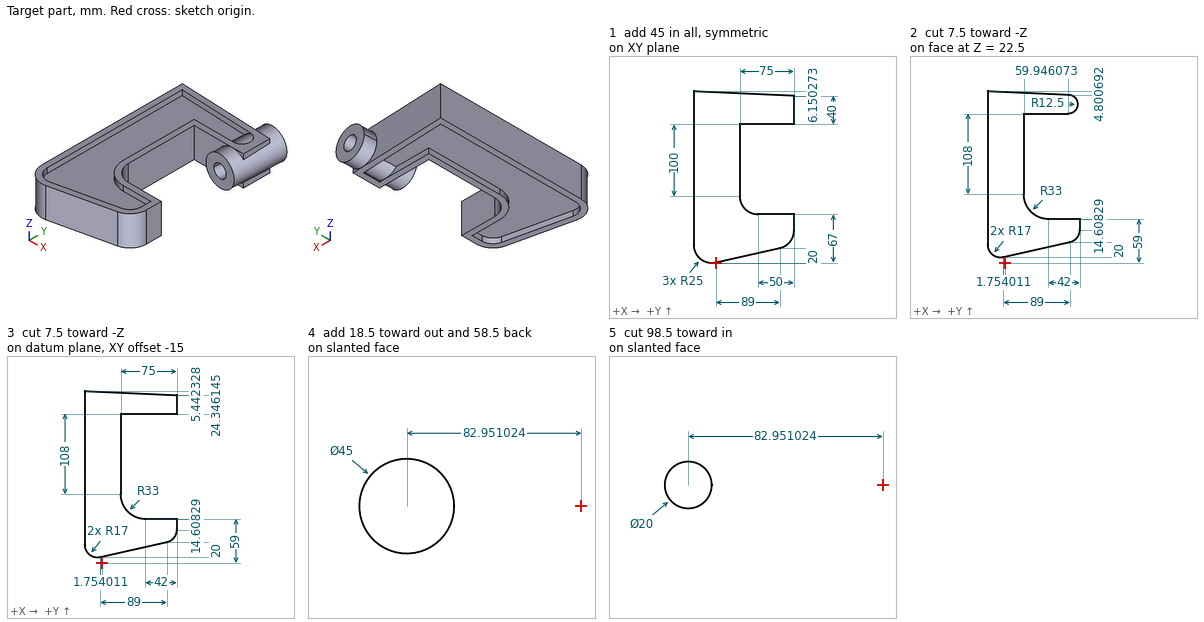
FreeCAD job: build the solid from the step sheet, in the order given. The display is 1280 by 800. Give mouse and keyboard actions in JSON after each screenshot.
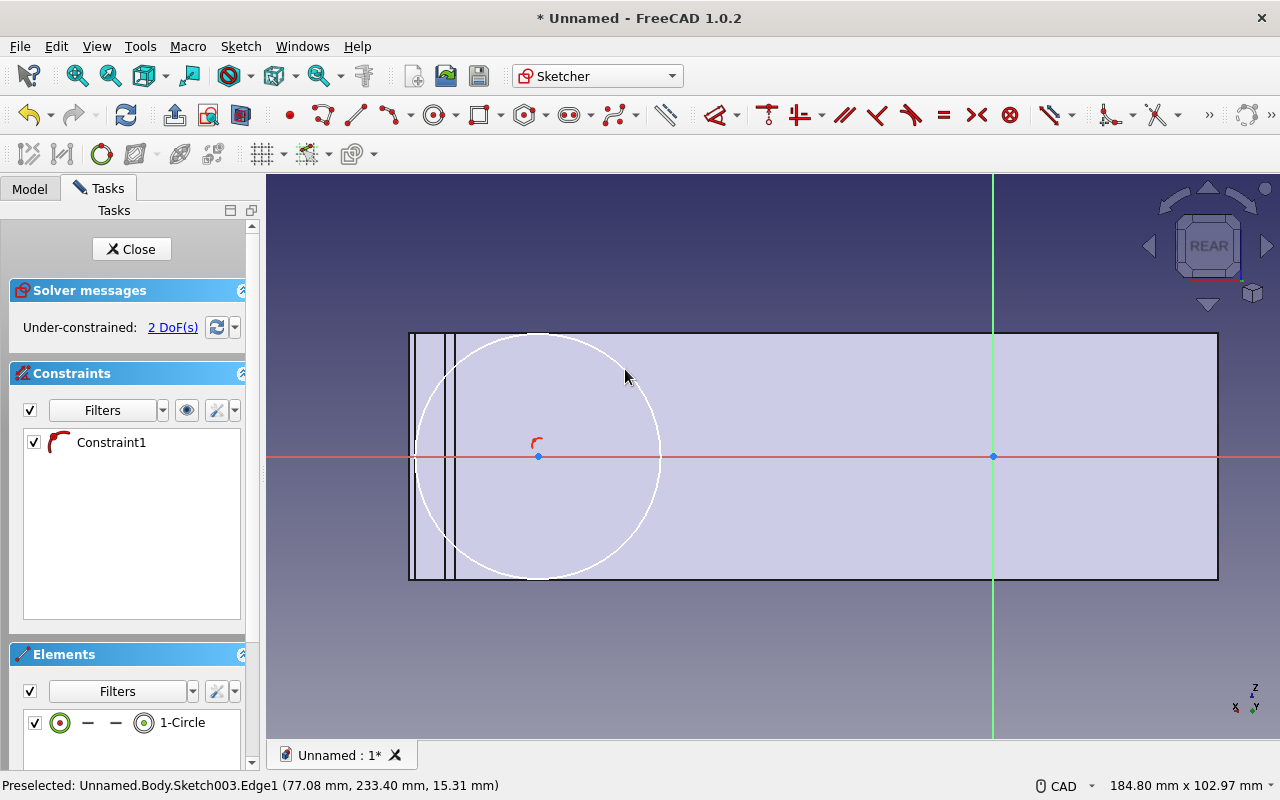
{"action": "left_click", "coordinate": [714, 116]}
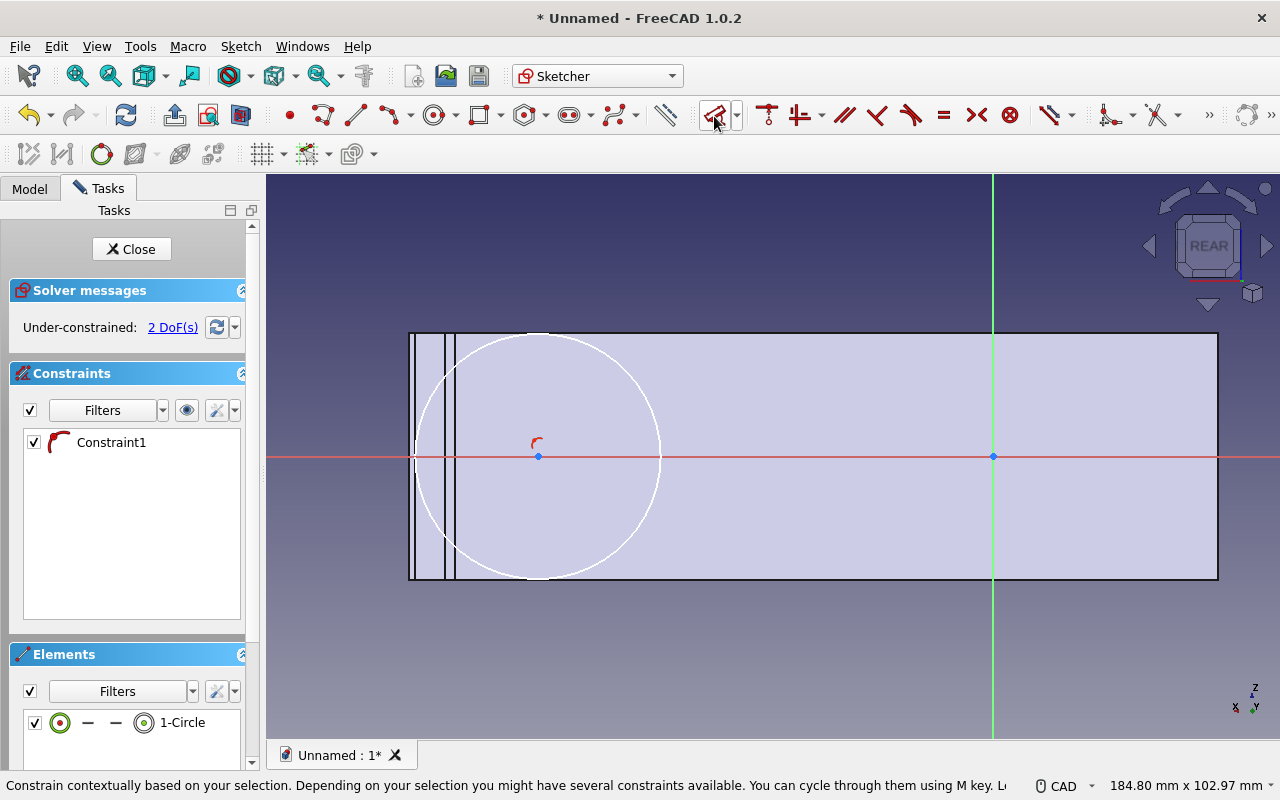
{"action": "left_click", "coordinate": [624, 369]}
{"action": "left_click", "coordinate": [646, 346]}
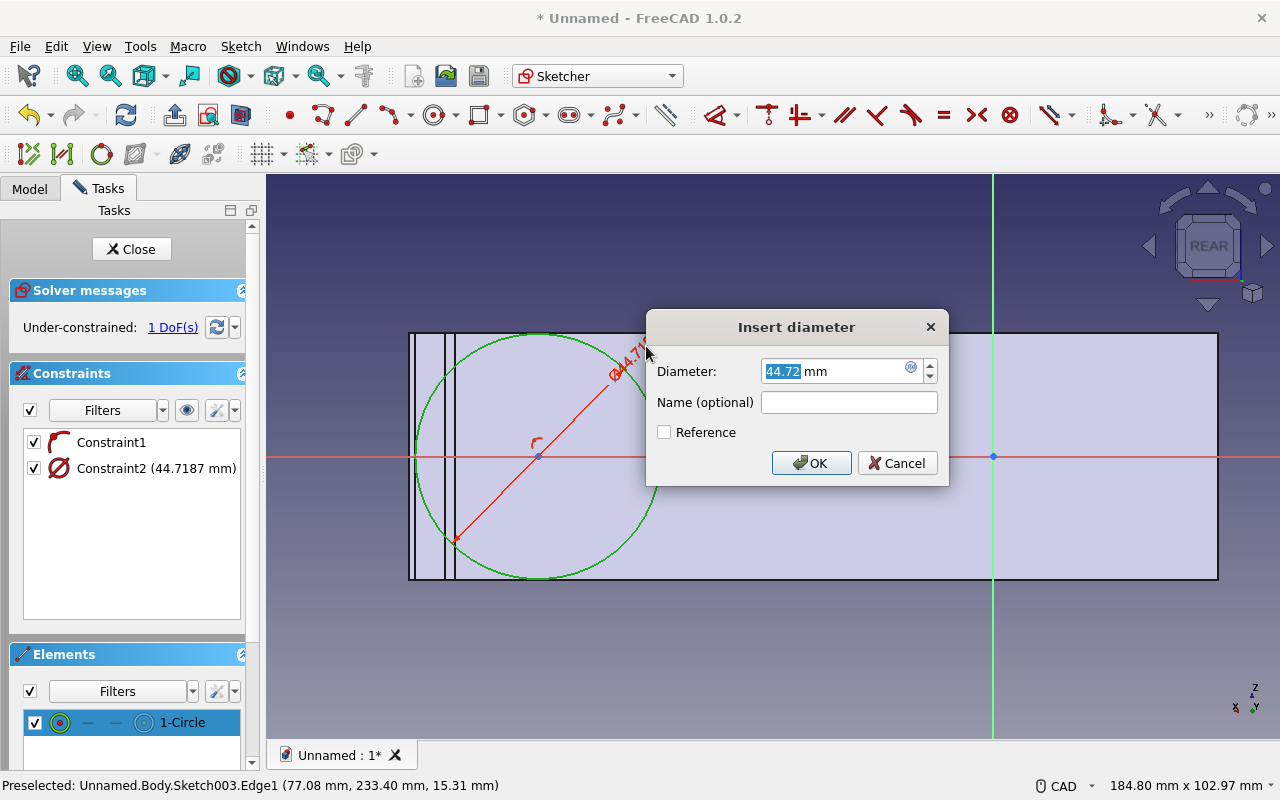
{"action": "type", "text": "45"}
{"action": "key", "text": "Return"}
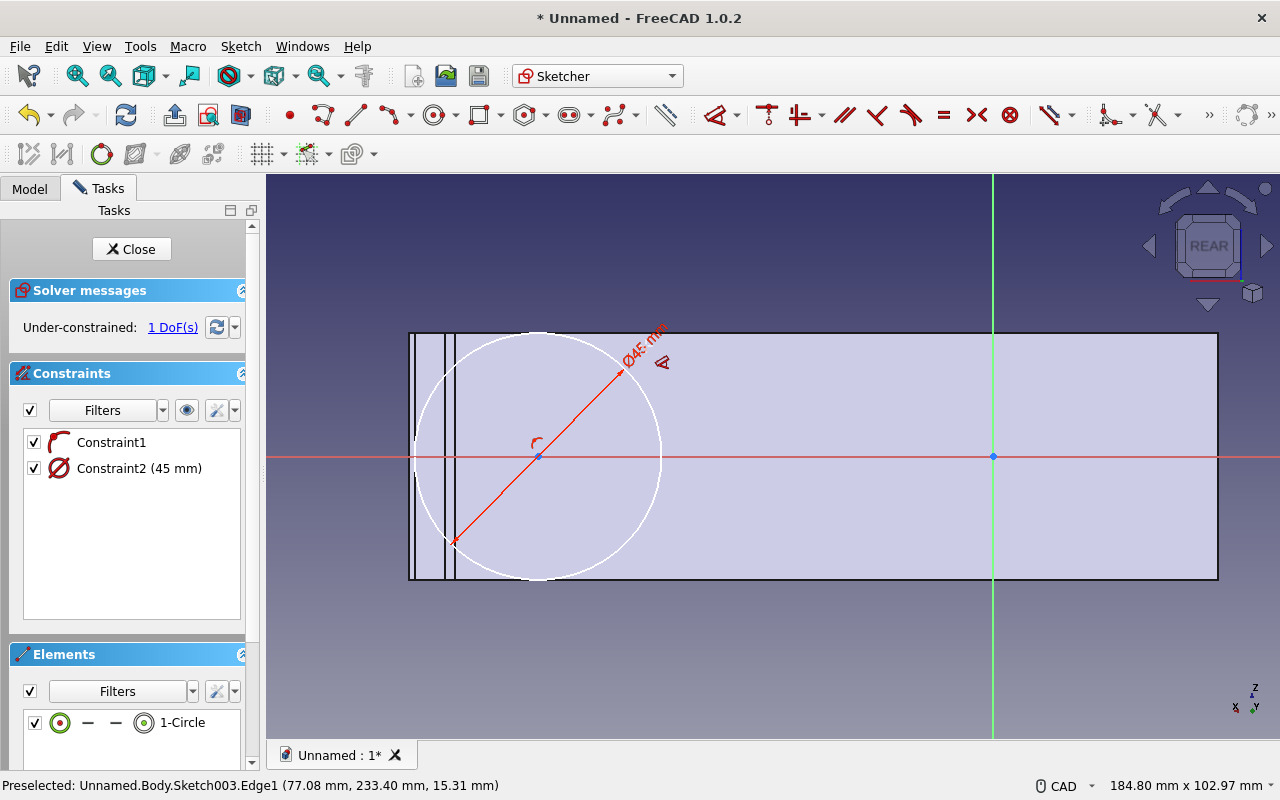
{"action": "left_click", "coordinate": [538, 456]}
{"action": "left_click", "coordinate": [766, 490]}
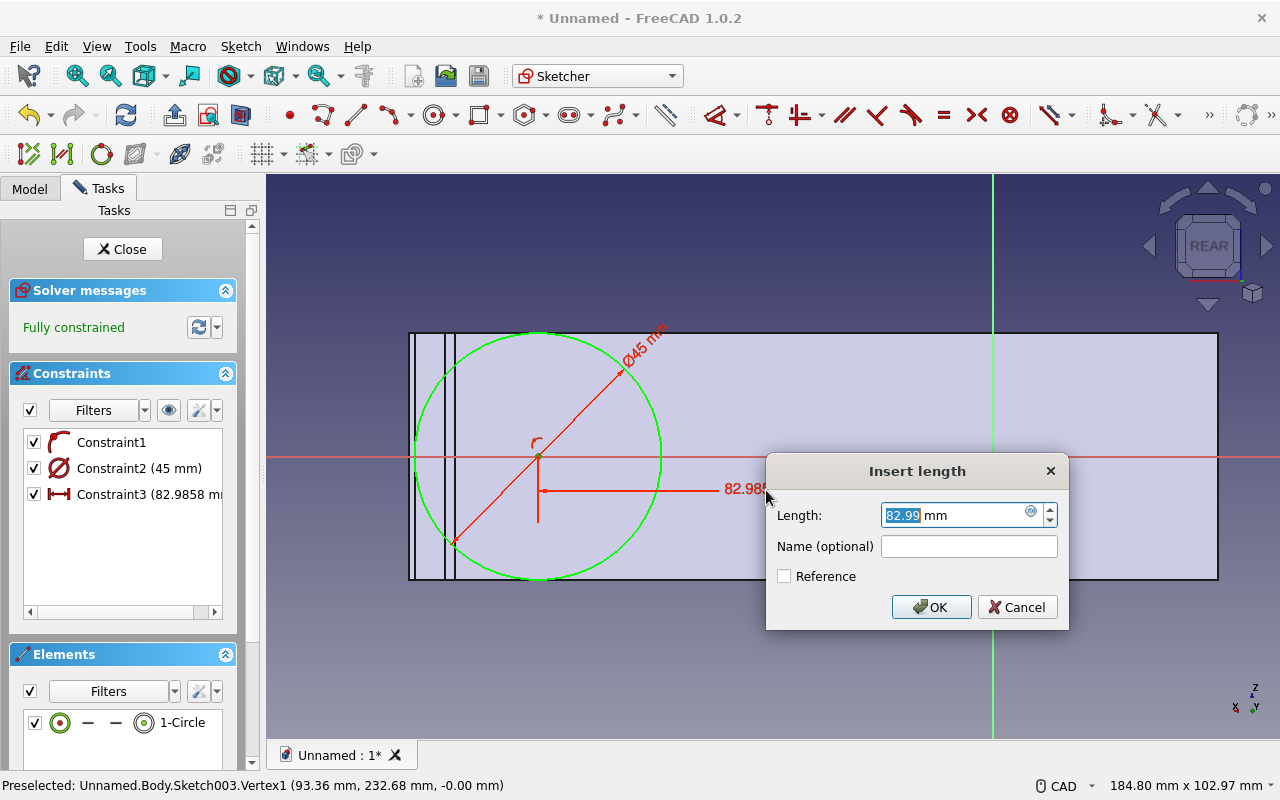
{"action": "type", "text": "82.951024"}
{"action": "key", "text": "Return"}
{"action": "key", "text": "Escape"}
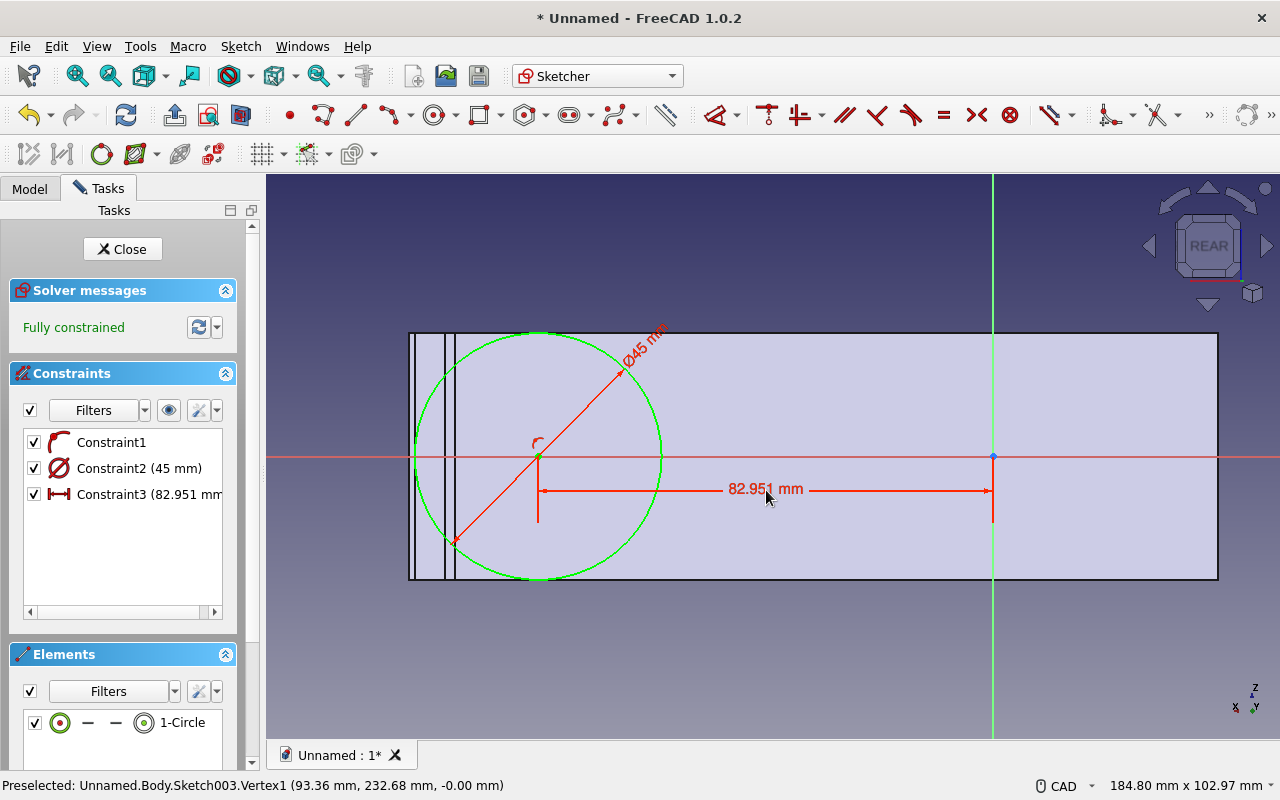
{"action": "left_click", "coordinate": [123, 249]}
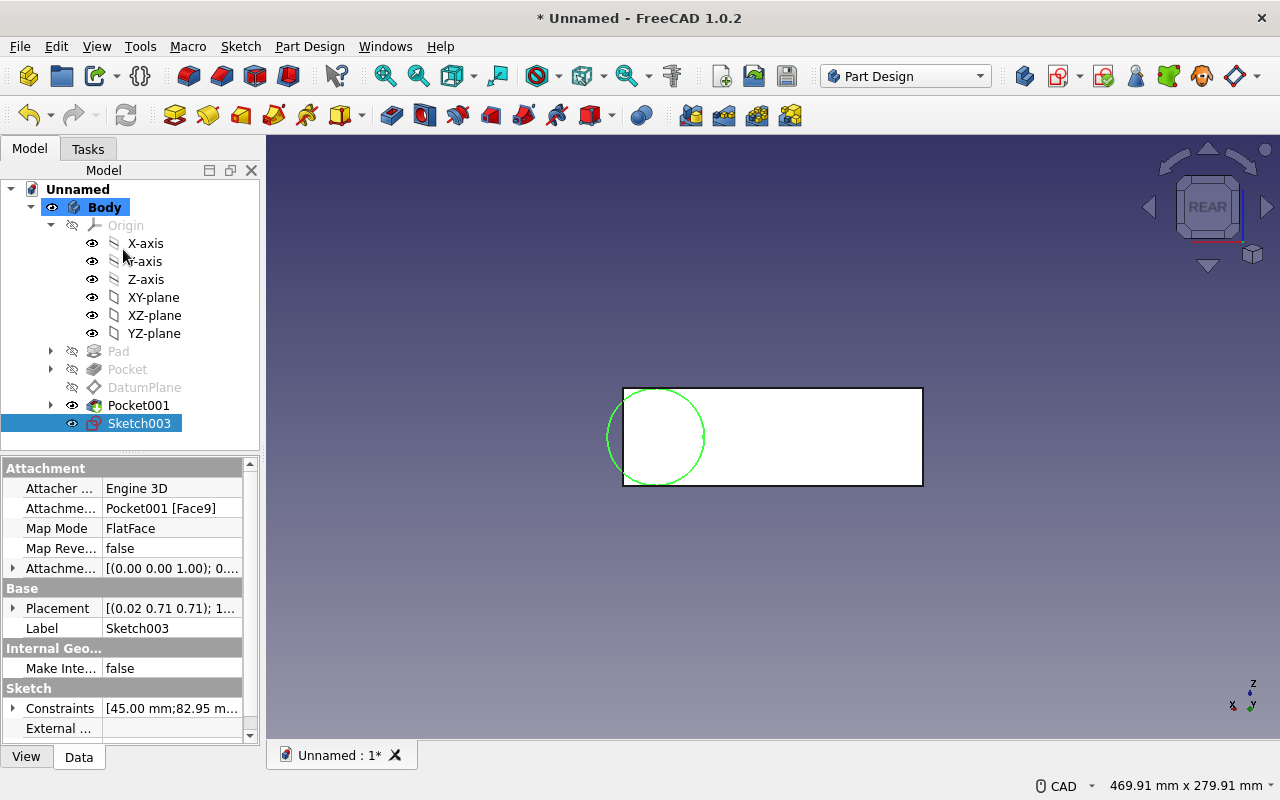
{"action": "left_click", "coordinate": [175, 116]}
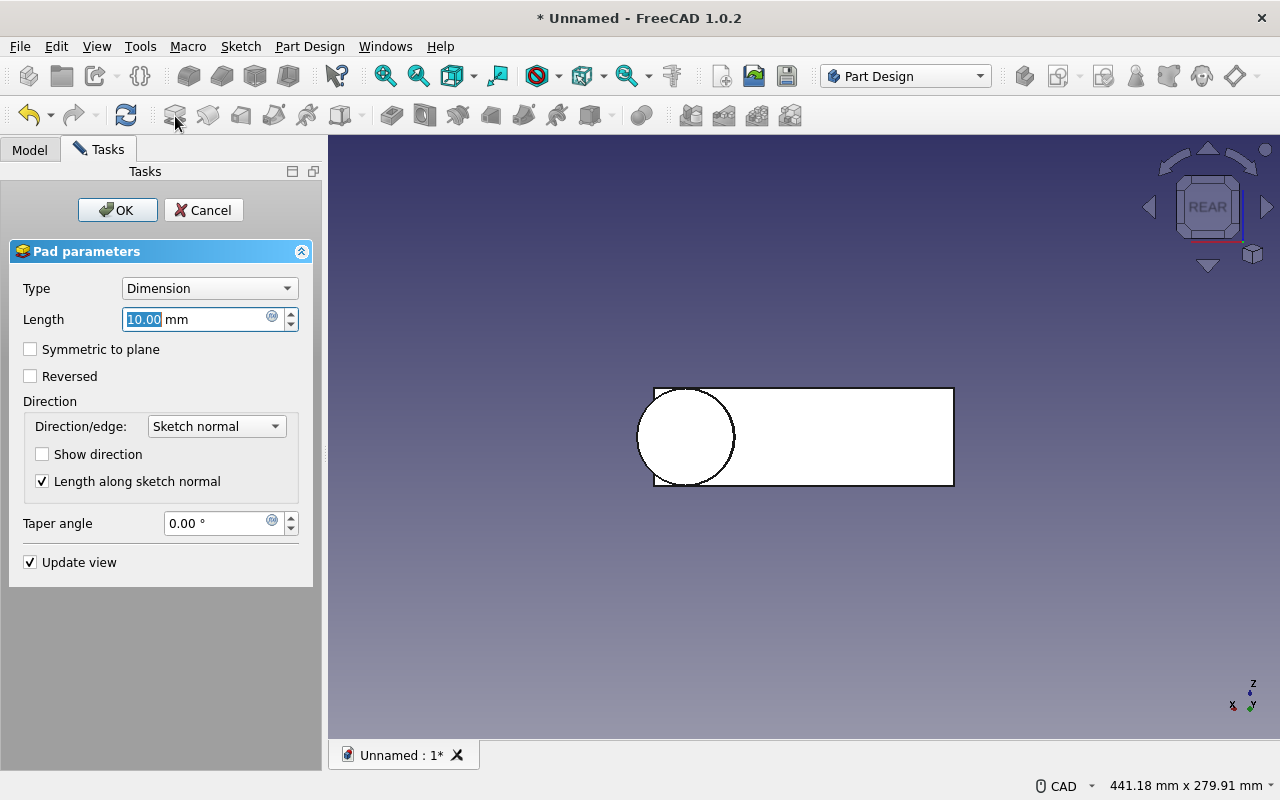
{"action": "left_click", "coordinate": [210, 288]}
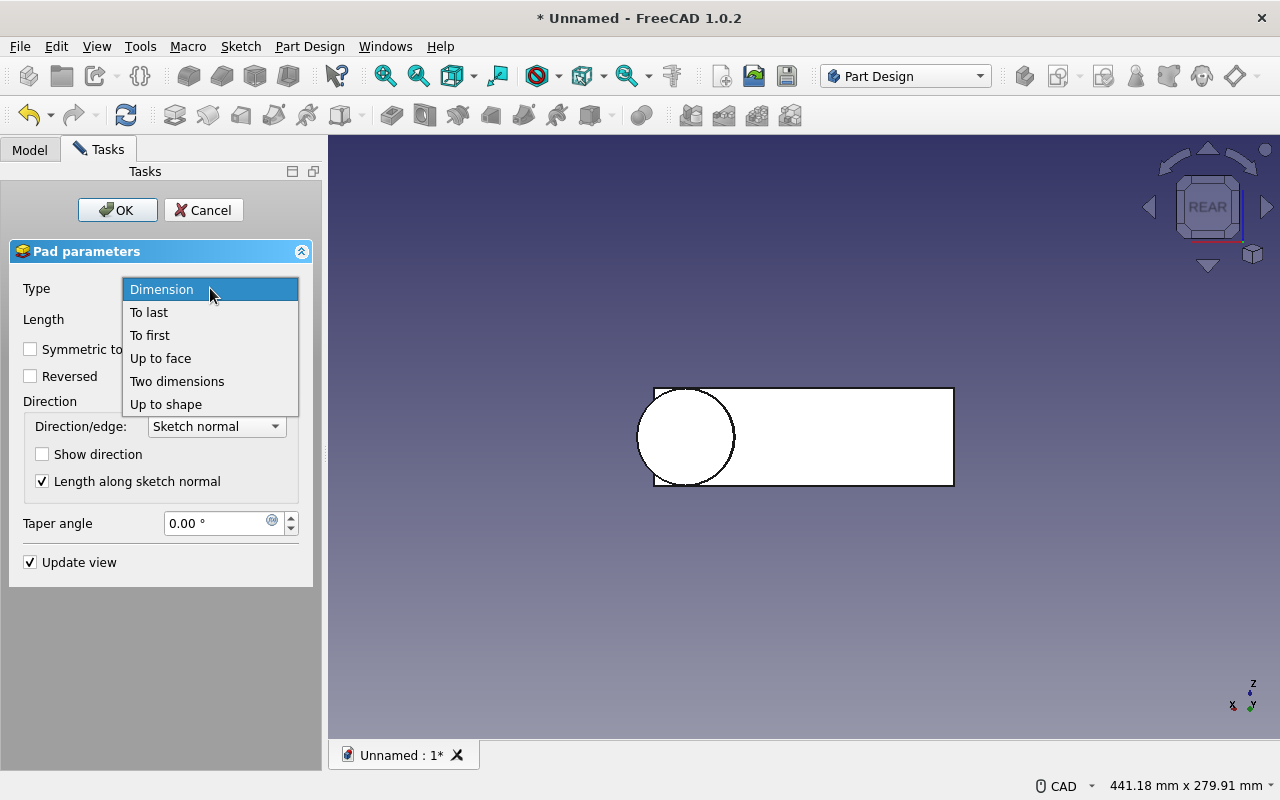
{"action": "left_click", "coordinate": [208, 382]}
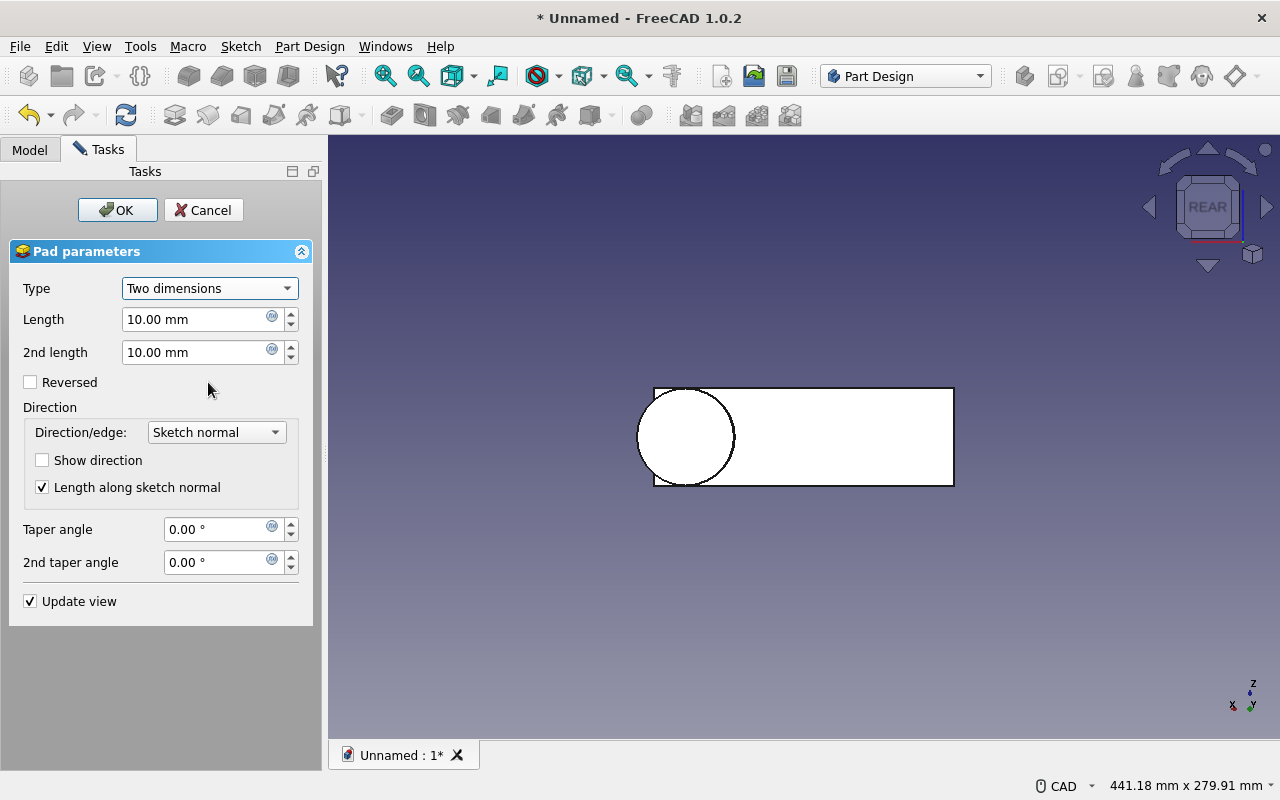
{"action": "triple_click", "coordinate": [204, 320]}